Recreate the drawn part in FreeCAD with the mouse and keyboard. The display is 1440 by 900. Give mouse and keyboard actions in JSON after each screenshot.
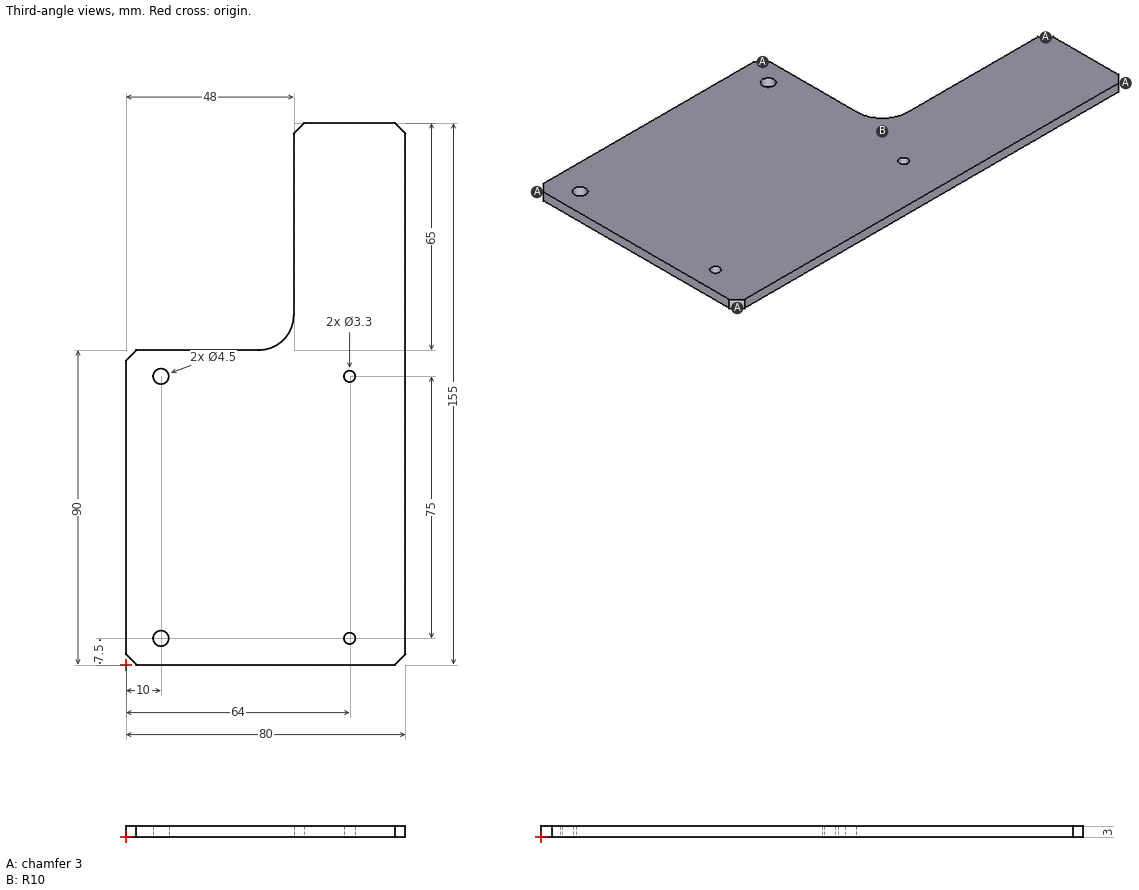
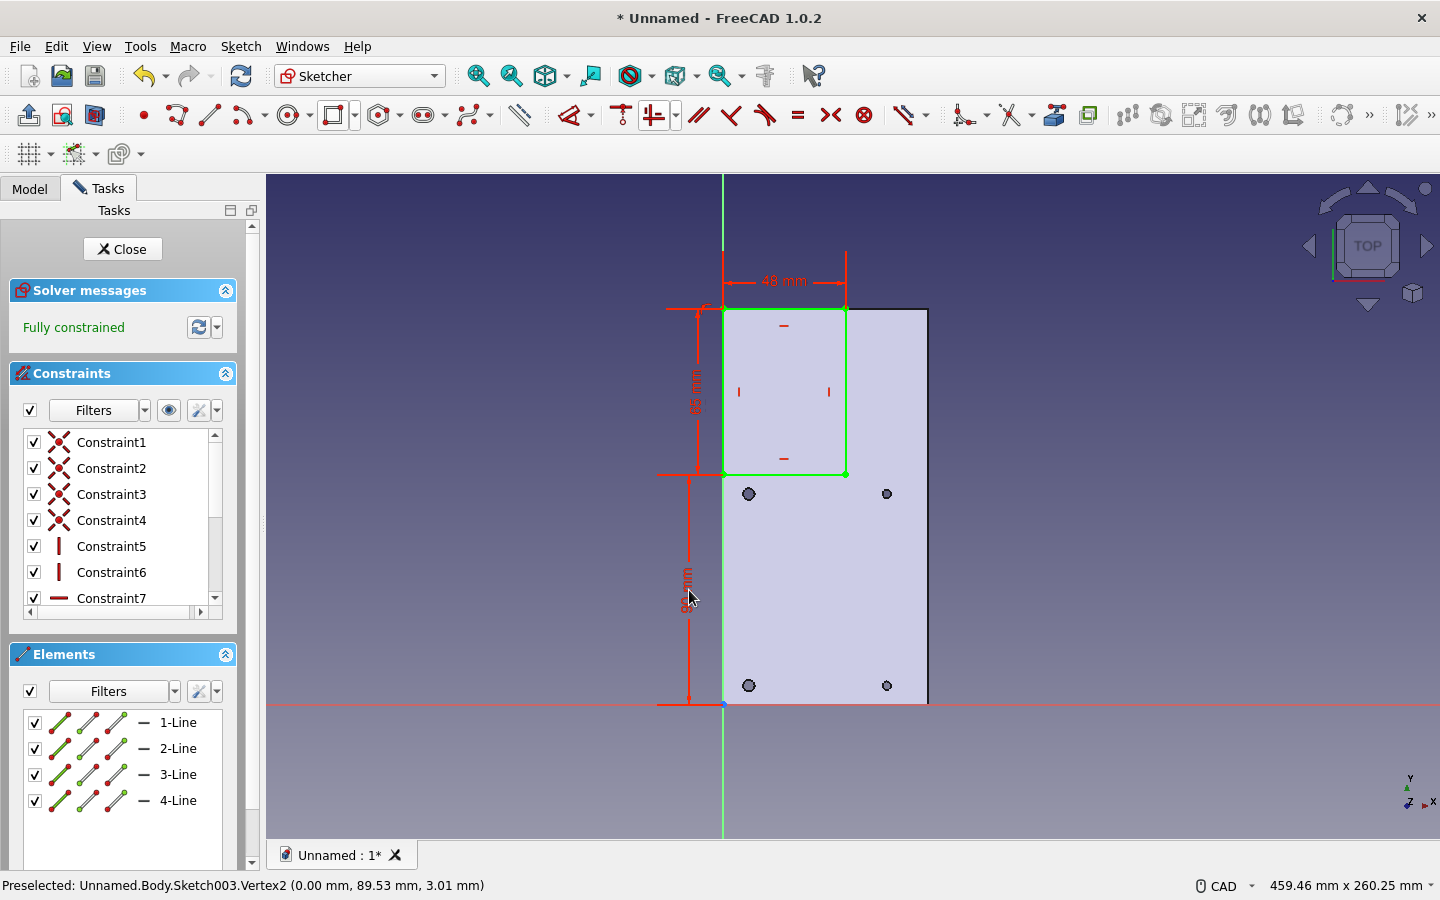
{"action": "left_click", "coordinate": [123, 249]}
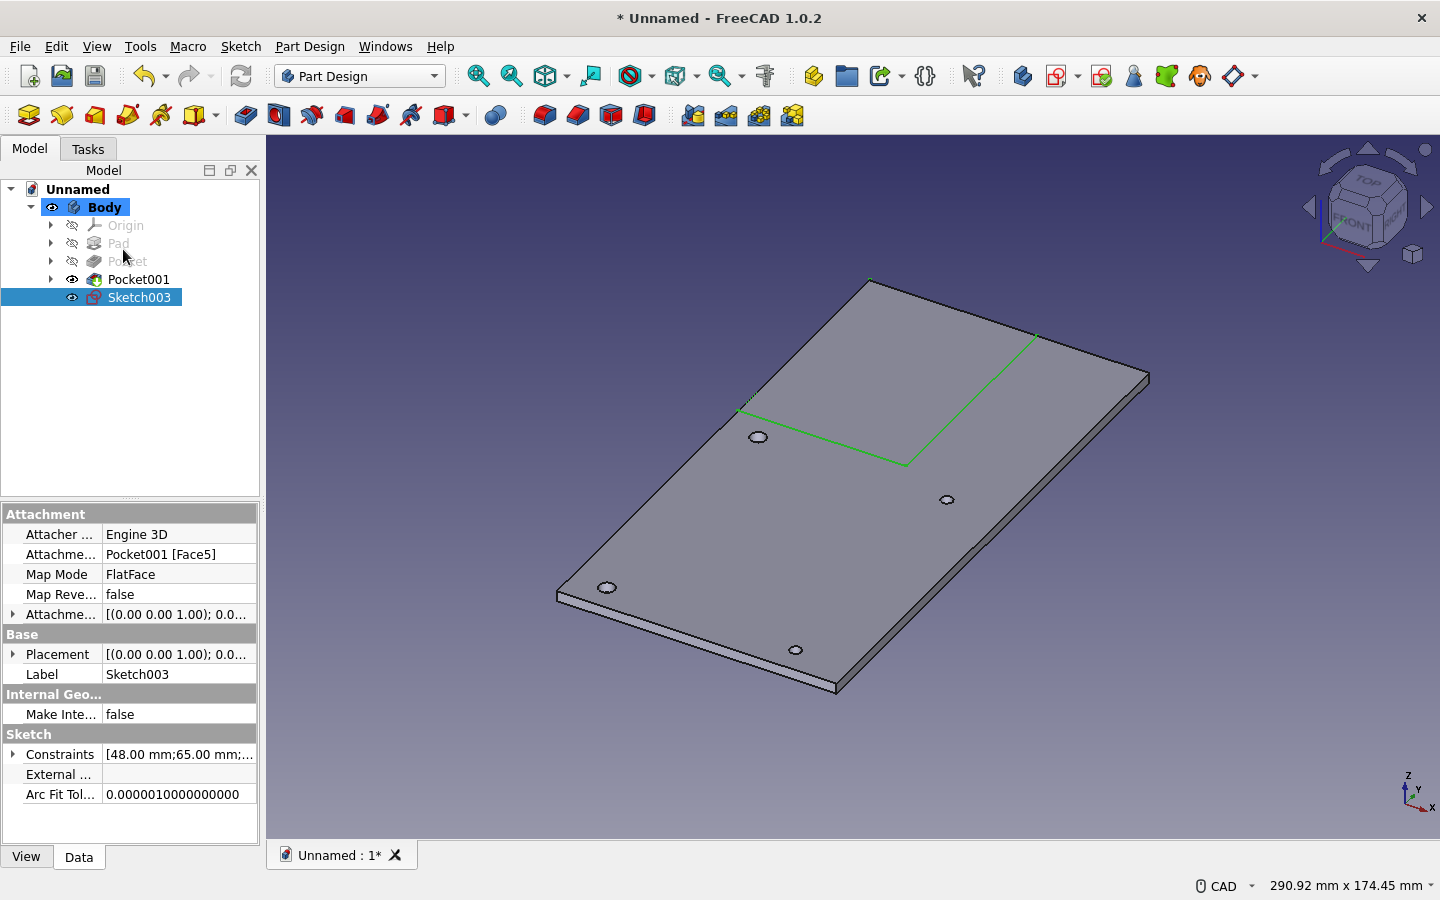
{"action": "left_click", "coordinate": [246, 116]}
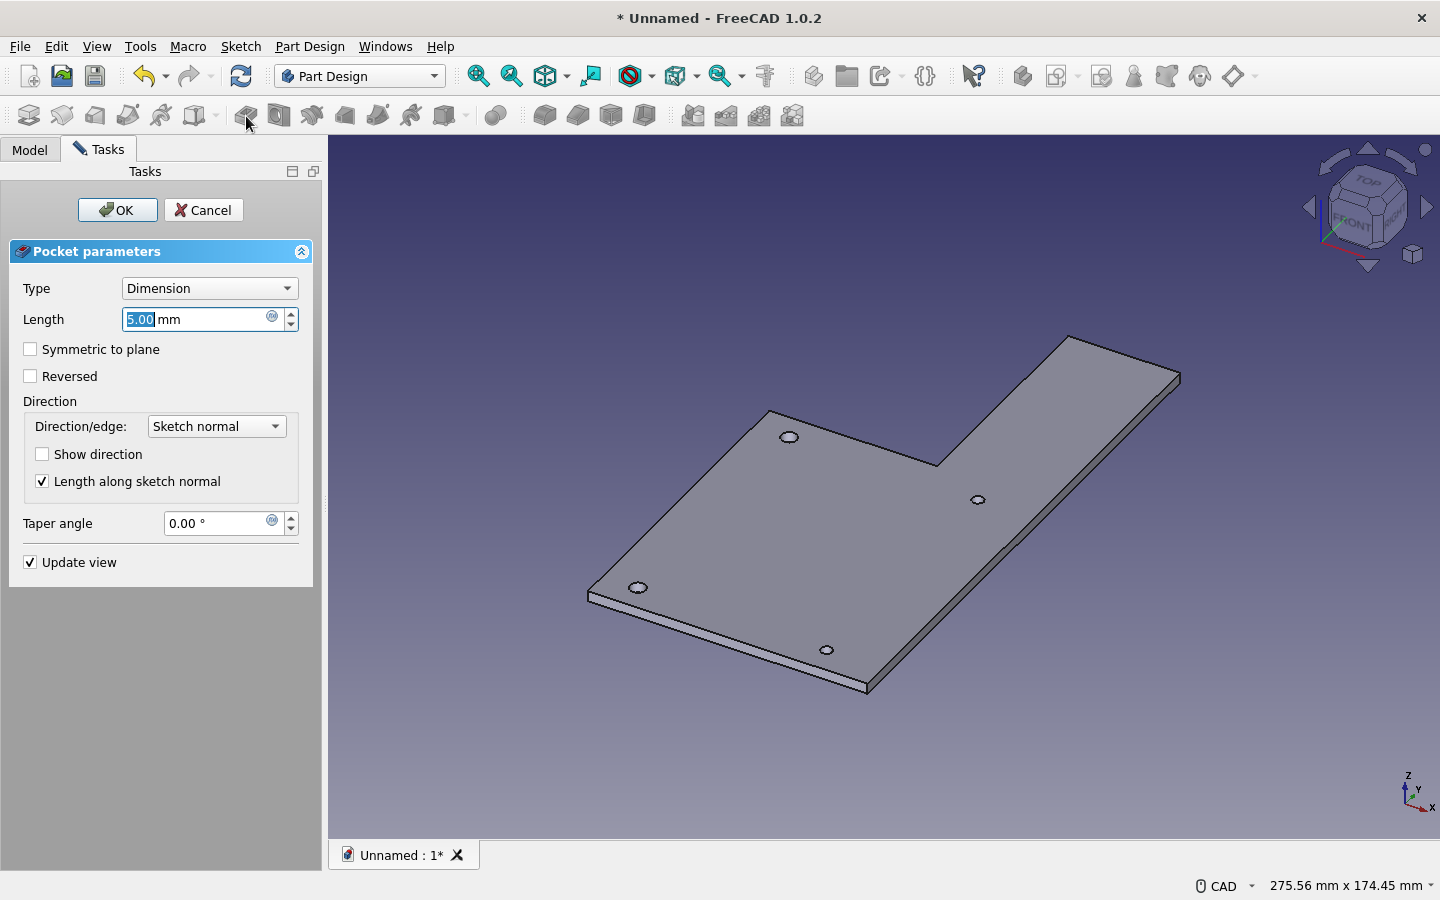
{"action": "left_click", "coordinate": [210, 288]}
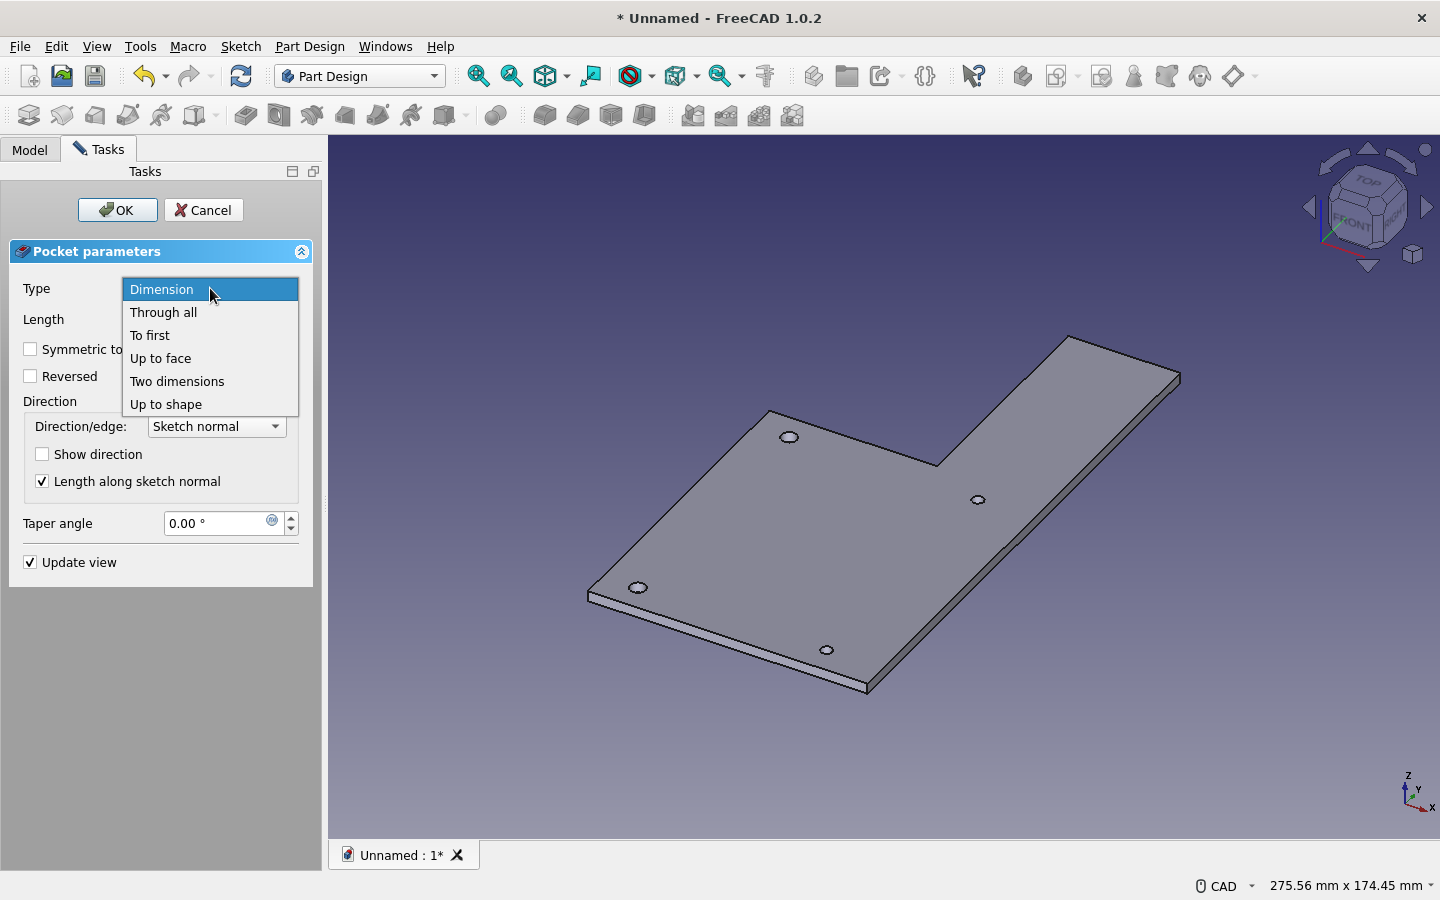
{"action": "left_click", "coordinate": [208, 312]}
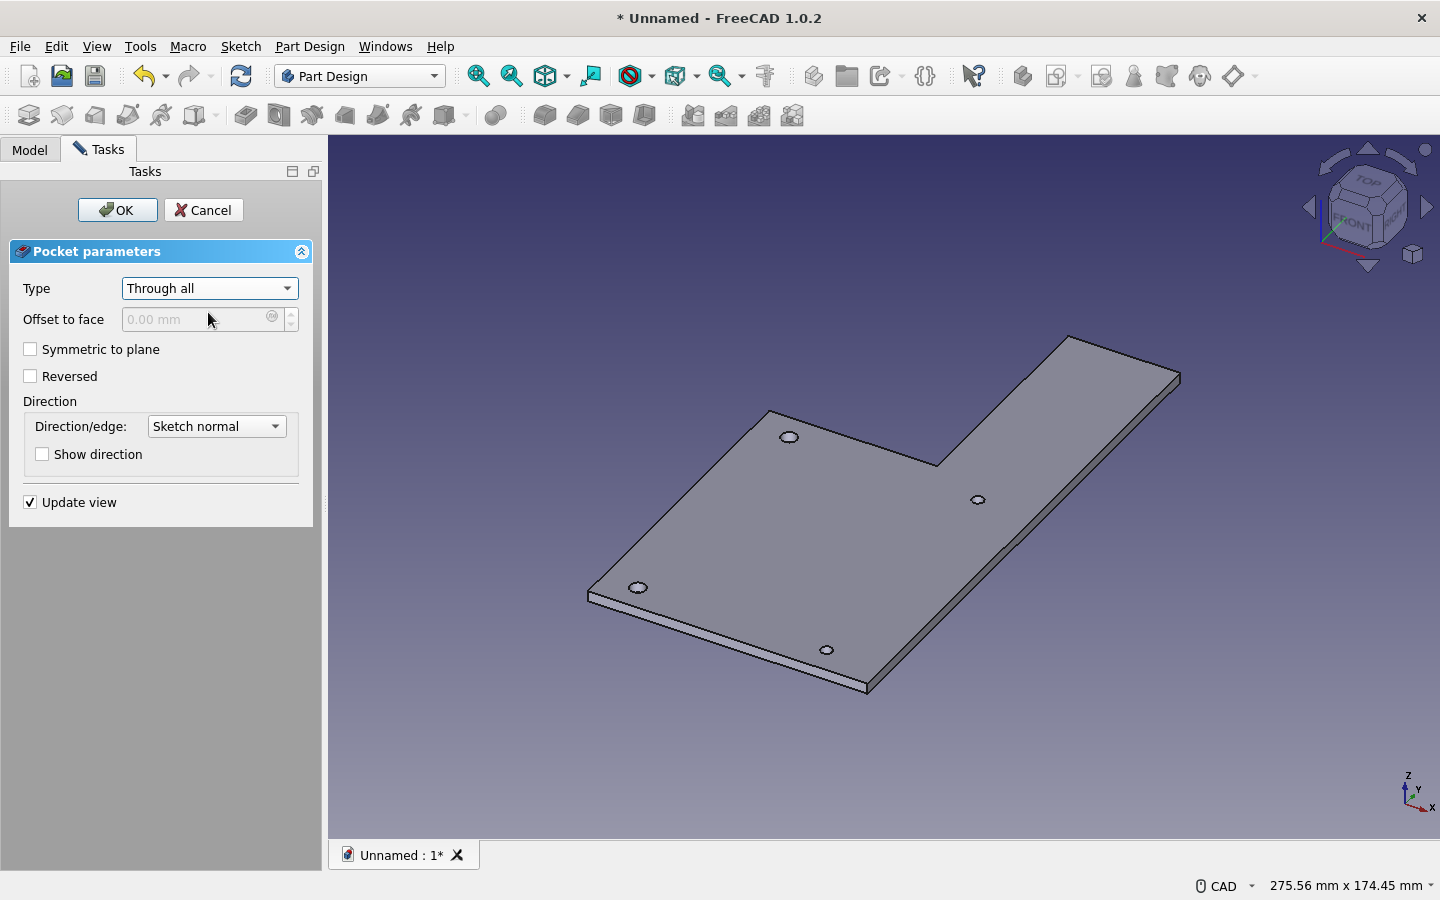
{"action": "left_click", "coordinate": [118, 210]}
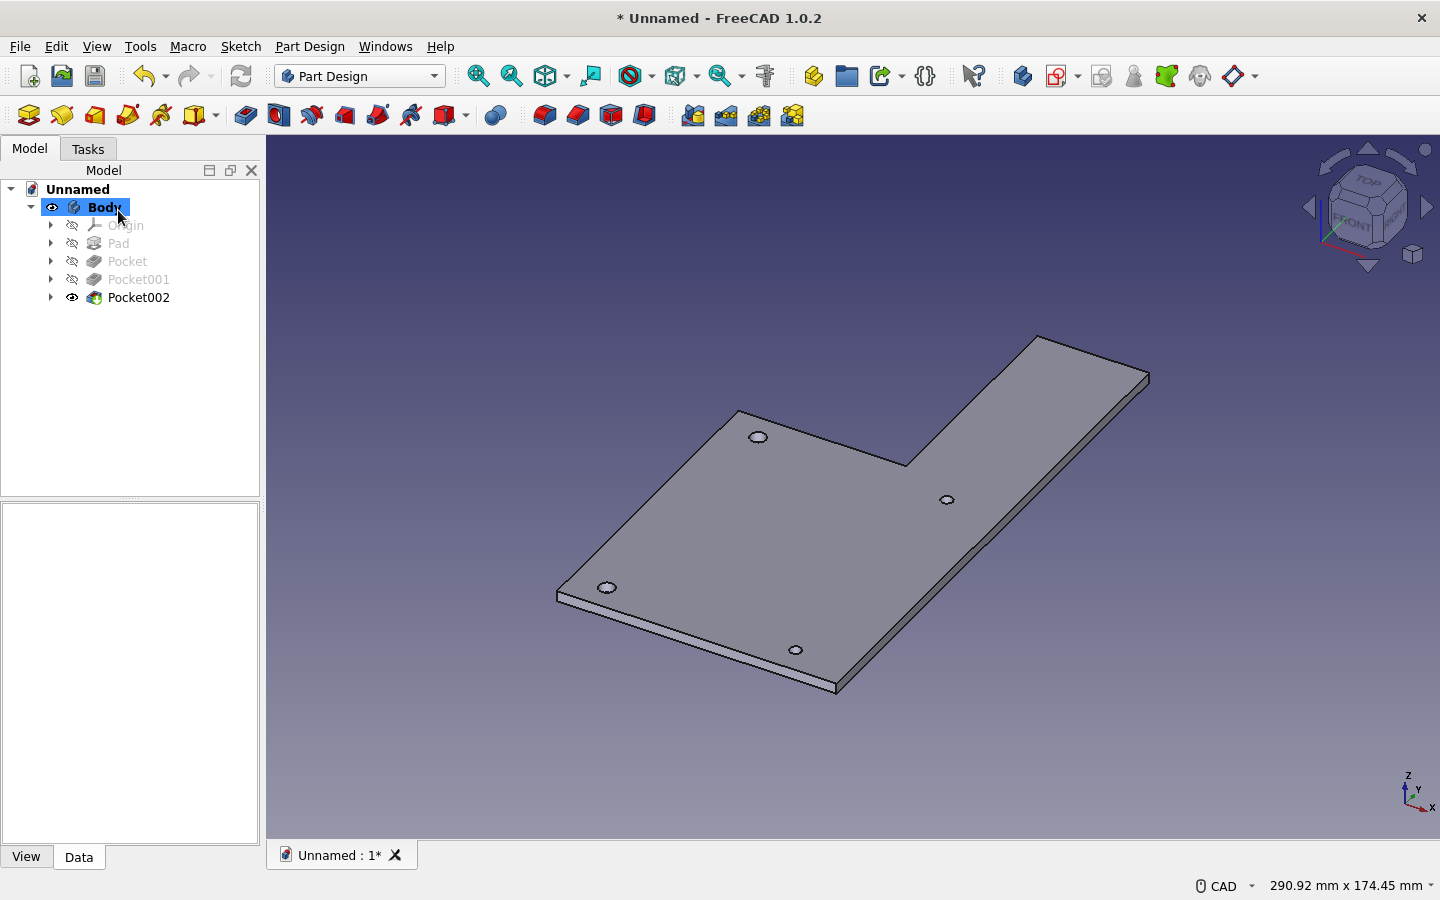
{"action": "left_click", "coordinate": [836, 689]}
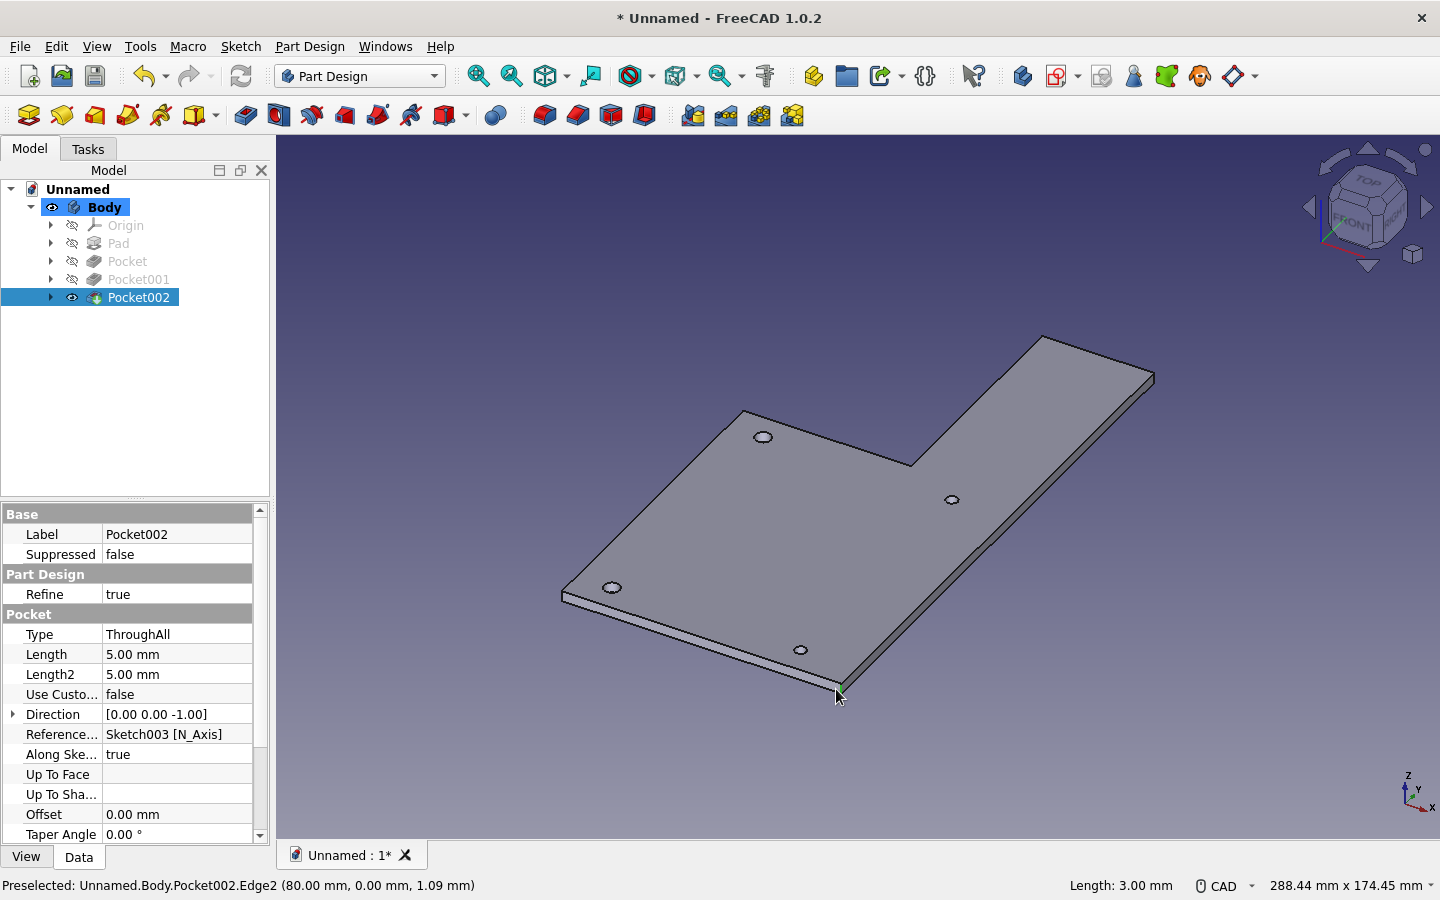
{"action": "scroll", "coordinate": [1042, 340], "scroll_direction": "up", "scroll_amount": 6}